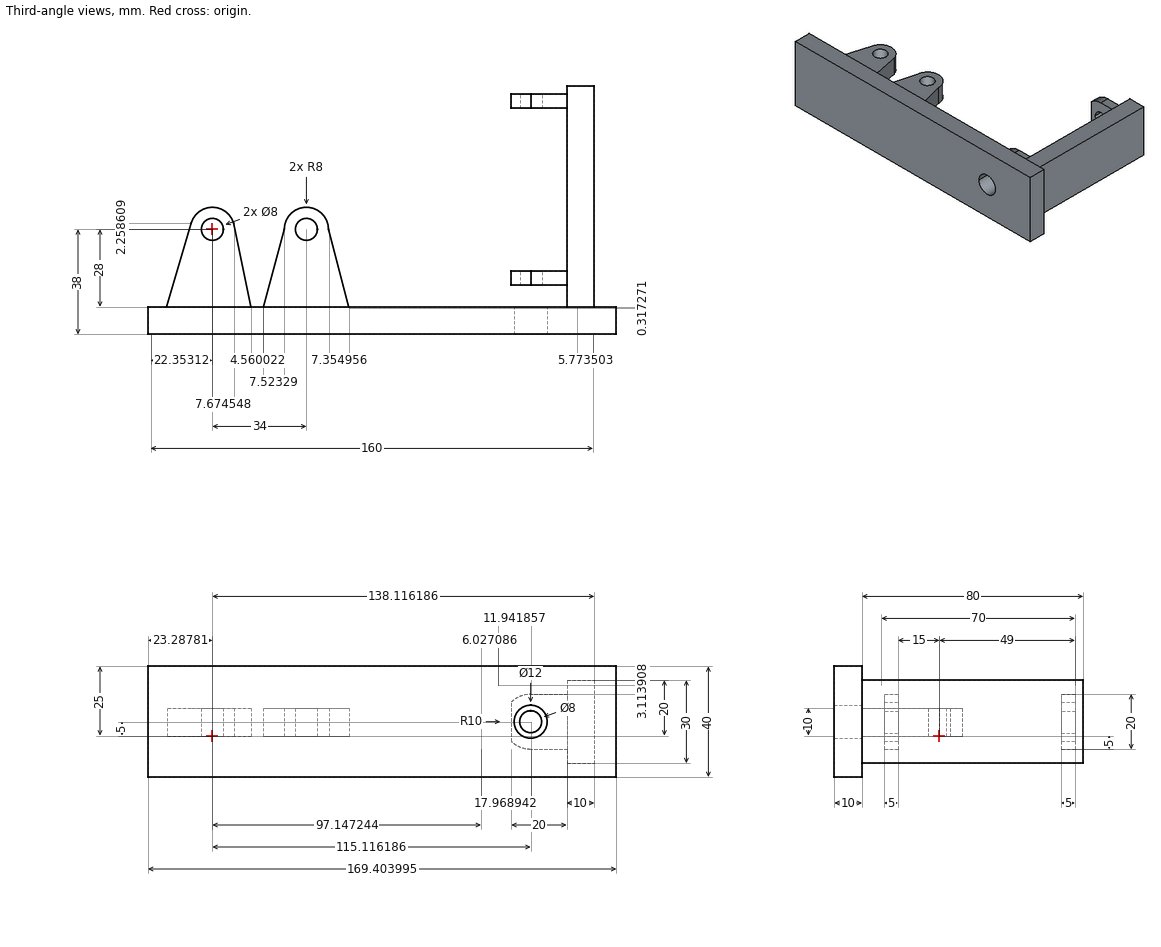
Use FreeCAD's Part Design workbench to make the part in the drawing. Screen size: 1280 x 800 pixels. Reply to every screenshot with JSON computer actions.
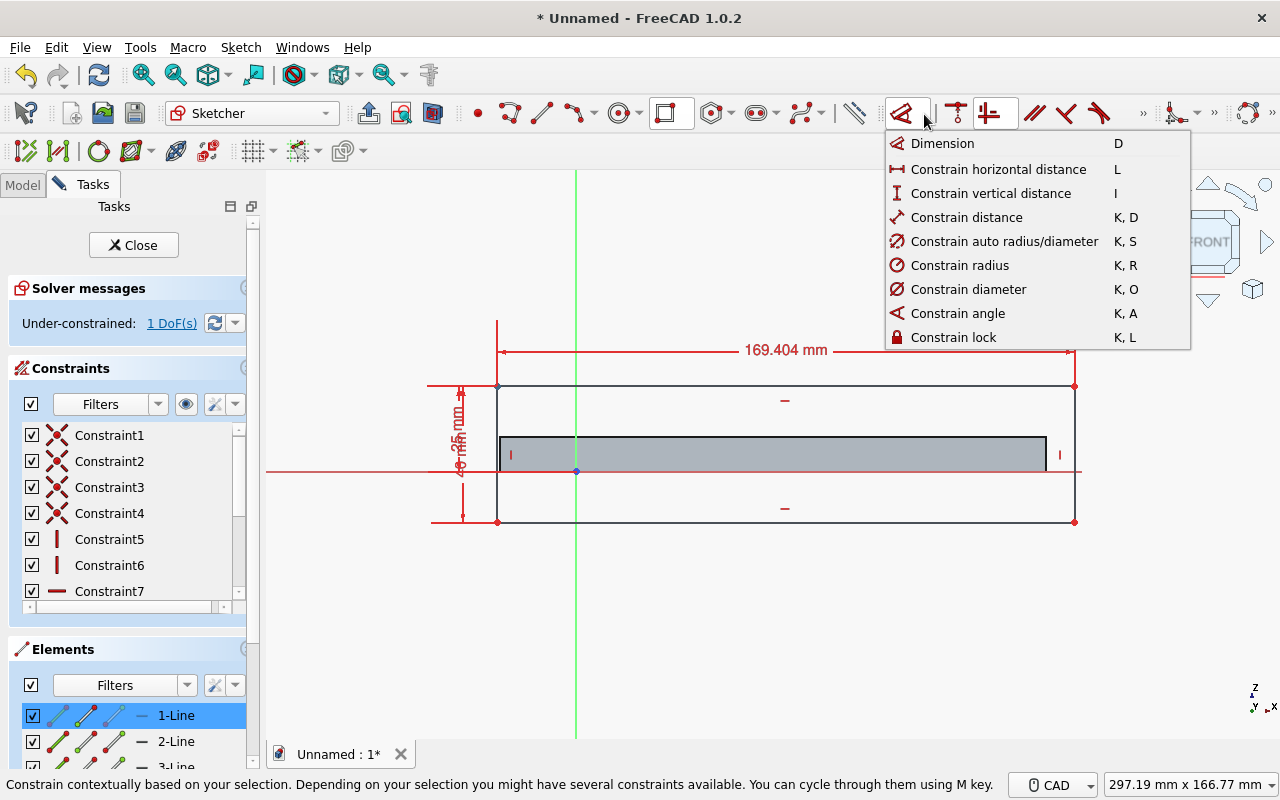
{"action": "left_click", "coordinate": [1038, 169]}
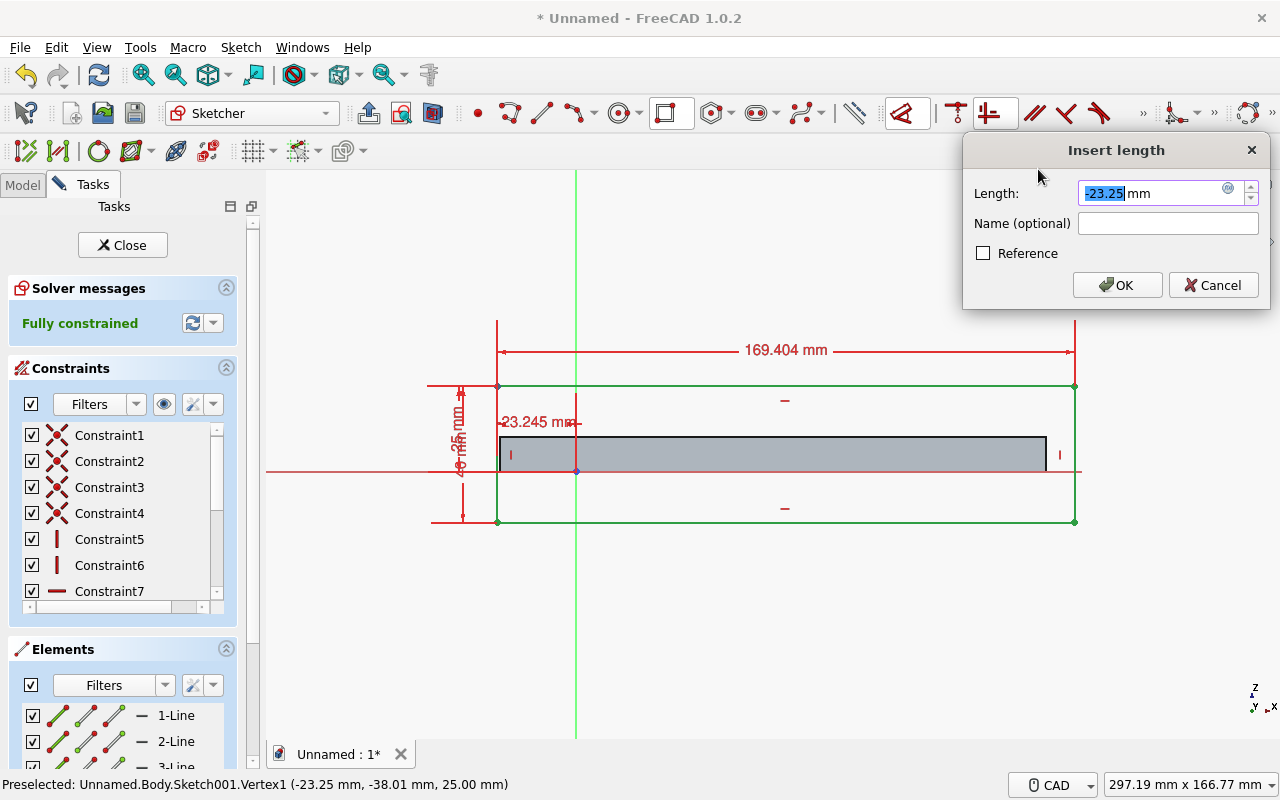
{"action": "type", "text": "-23.28781"}
{"action": "key", "text": "Return"}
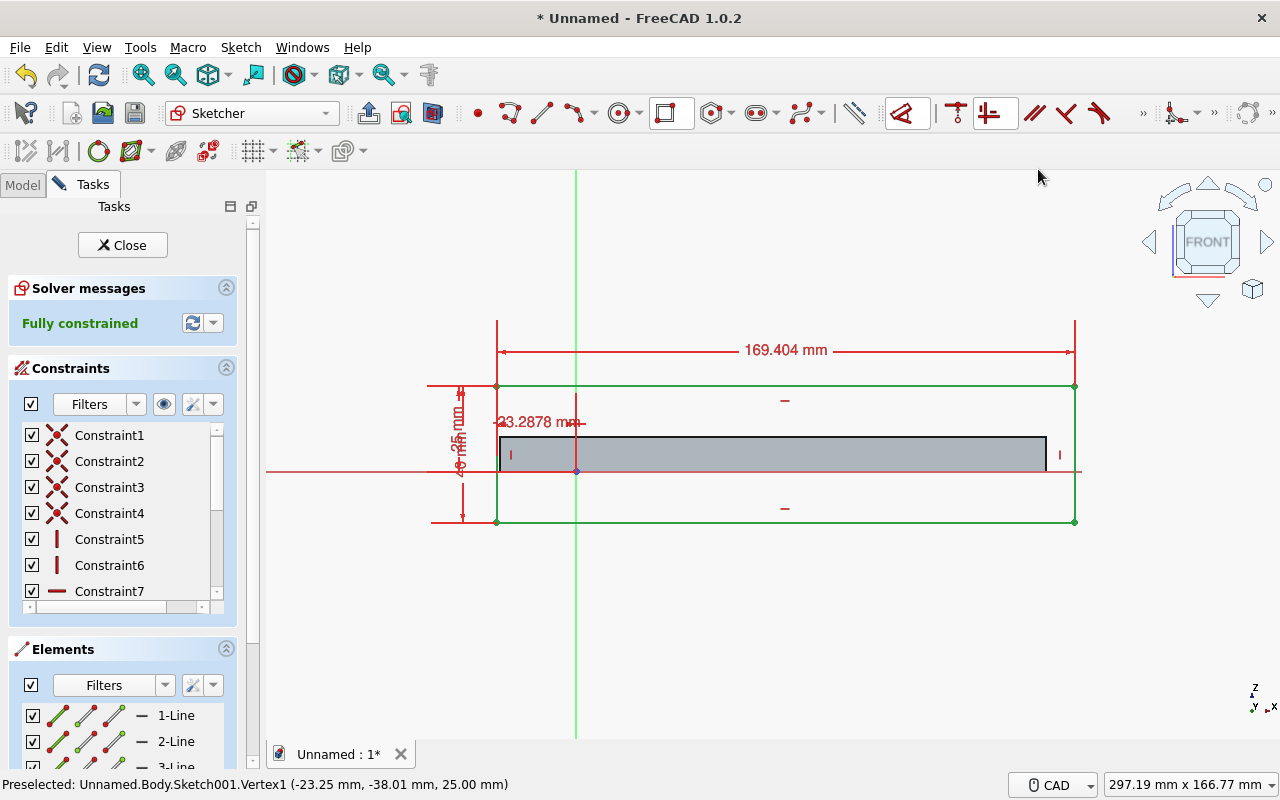
{"action": "left_click", "coordinate": [123, 245]}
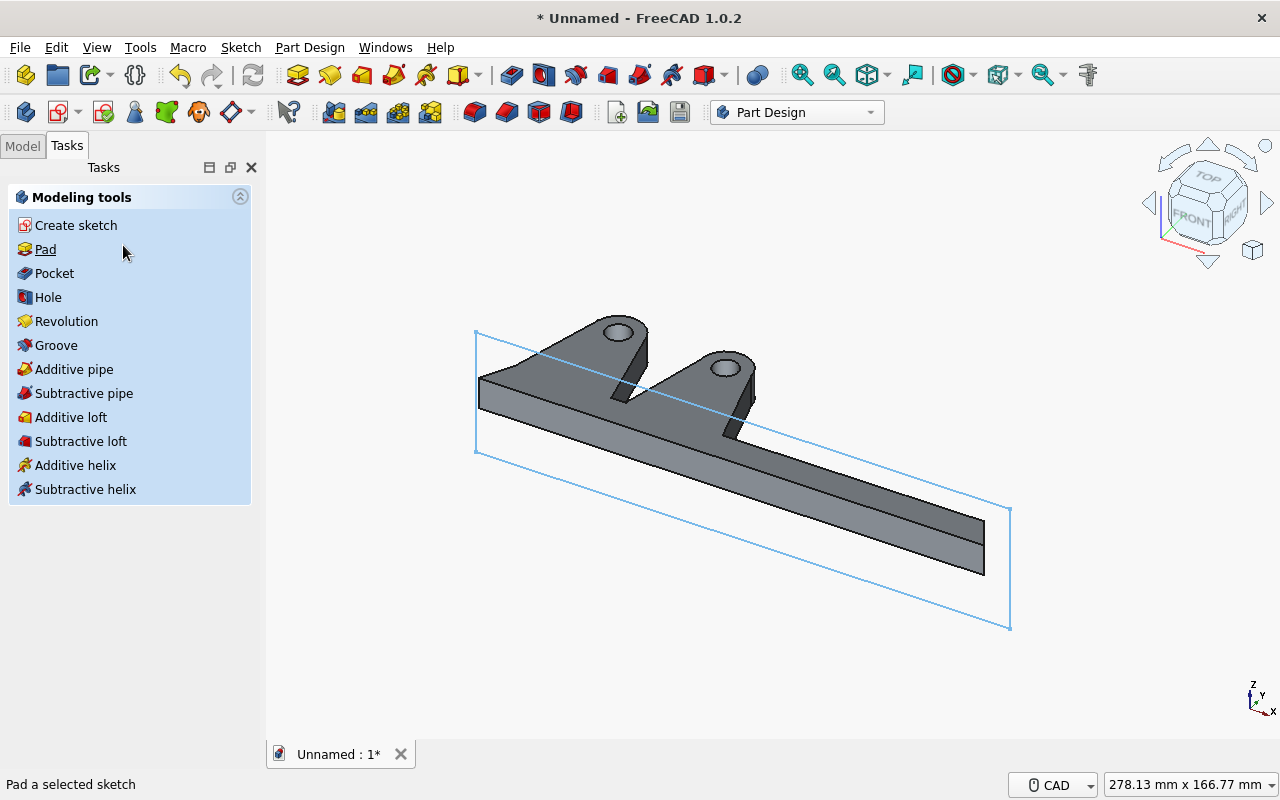
{"action": "left_click", "coordinate": [298, 76]}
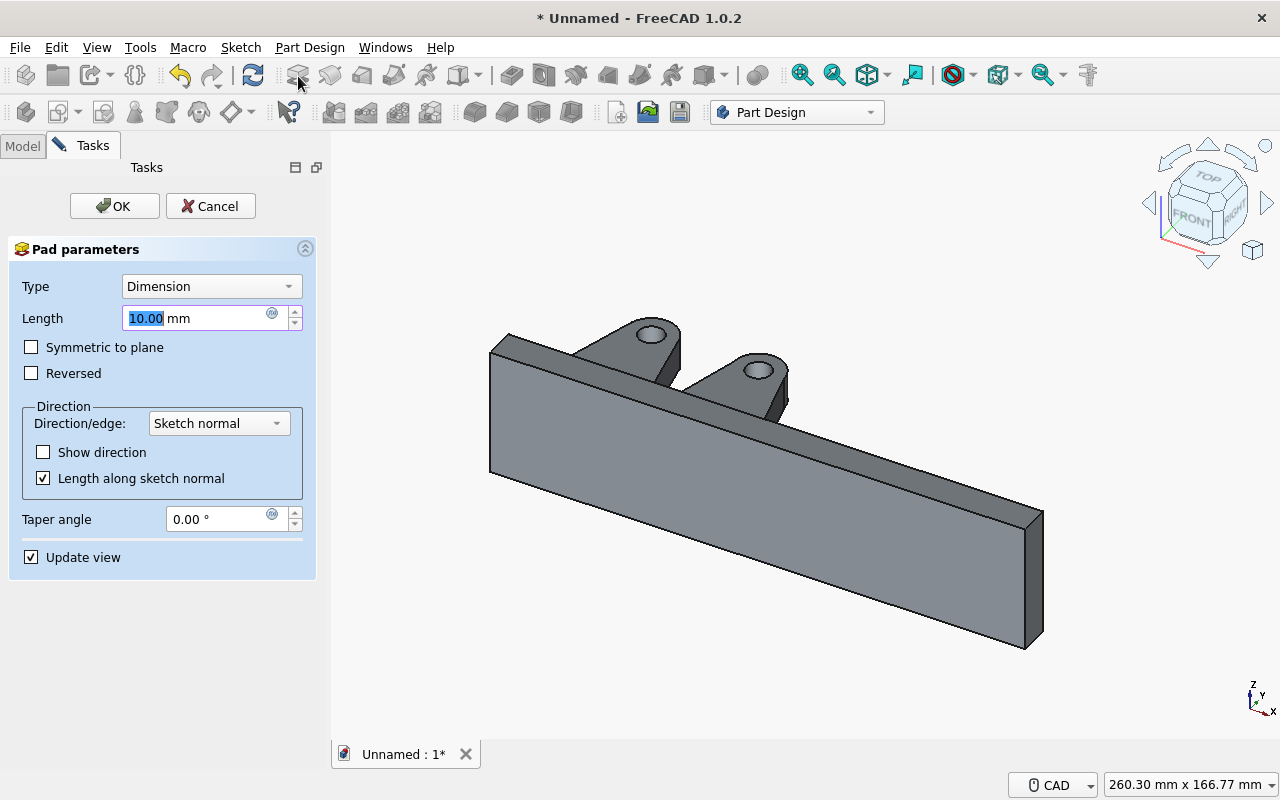
{"action": "type", "text": "10"}
{"action": "key", "text": "Tab"}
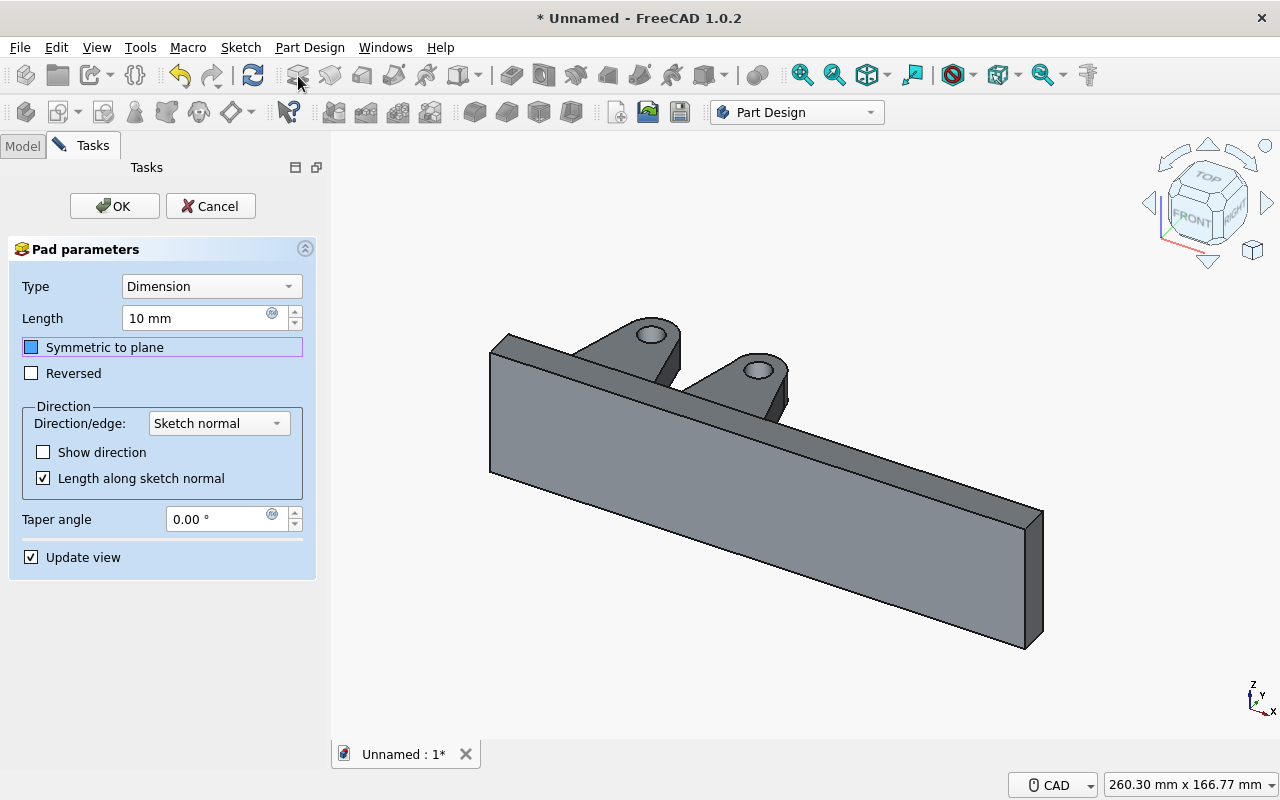
{"action": "left_click", "coordinate": [30, 373]}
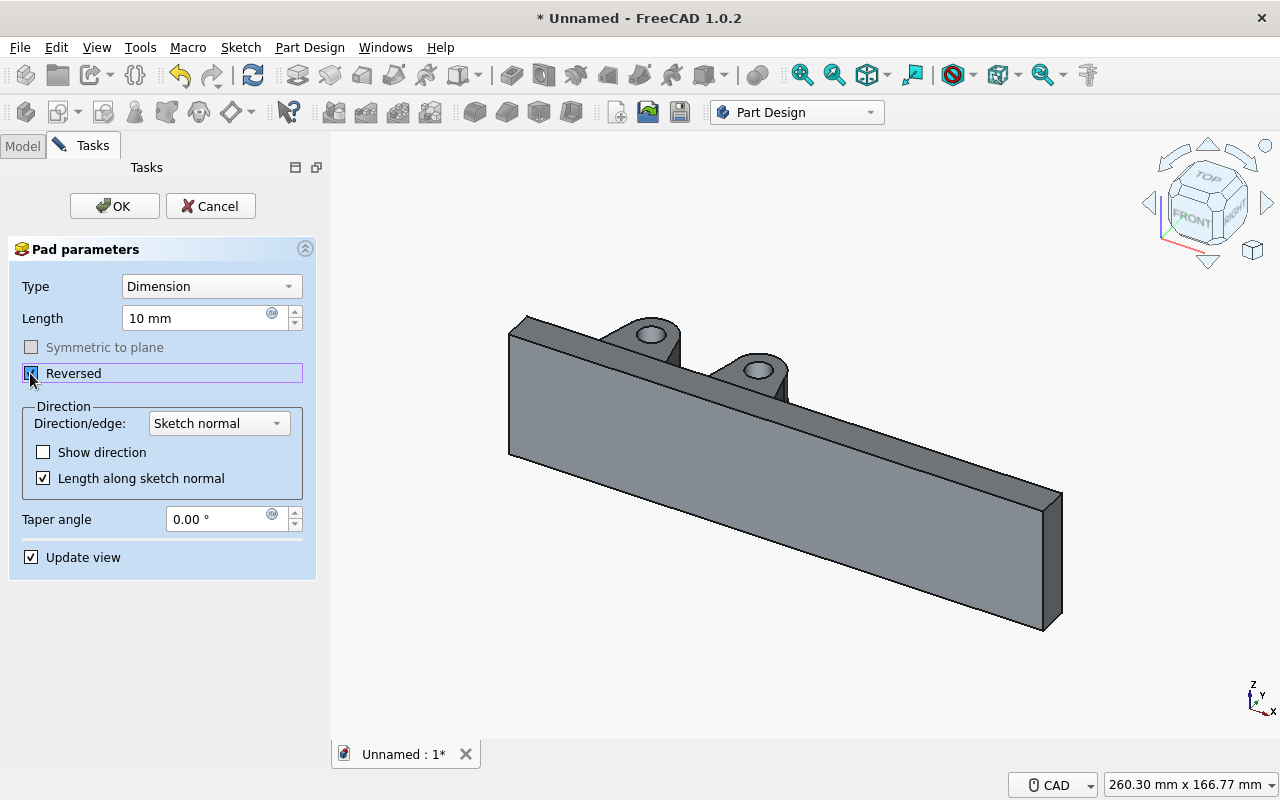
{"action": "left_click", "coordinate": [115, 206]}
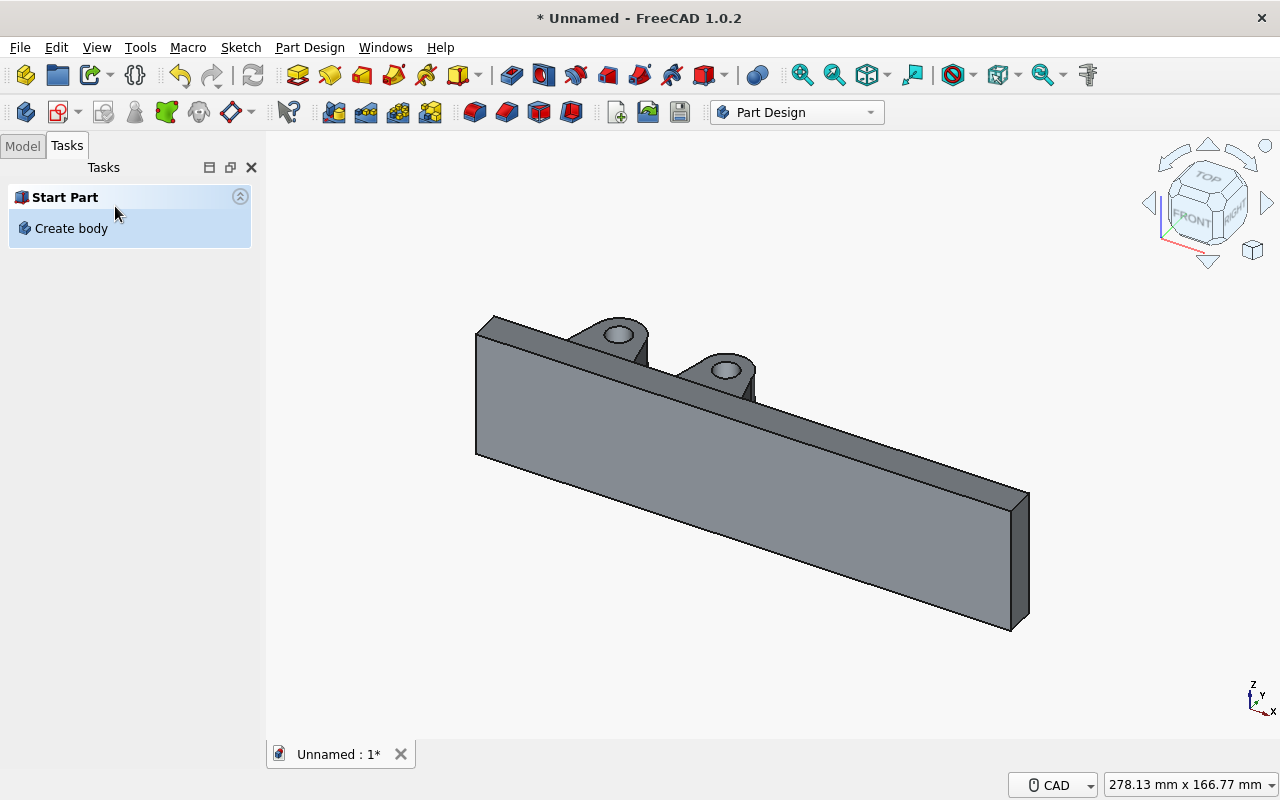
{"action": "key", "text": "4"}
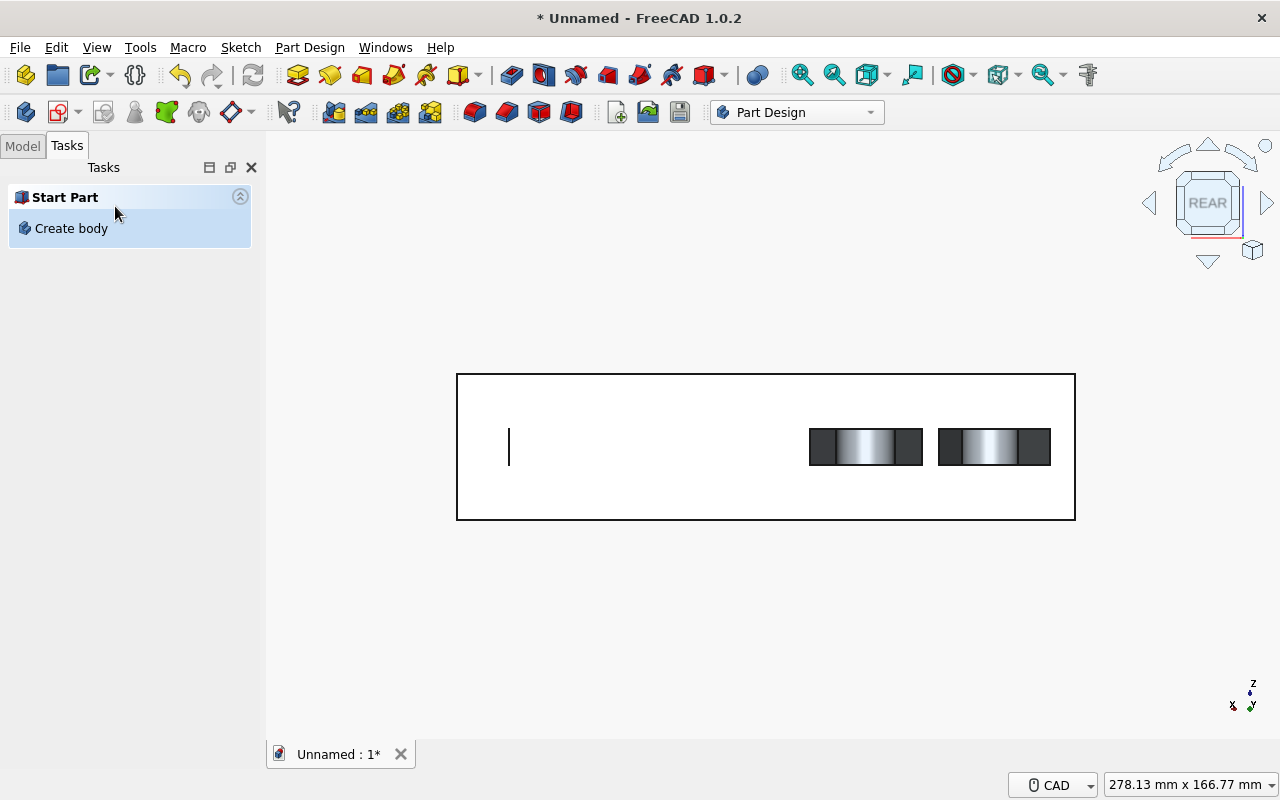
{"action": "left_click", "coordinate": [589, 446]}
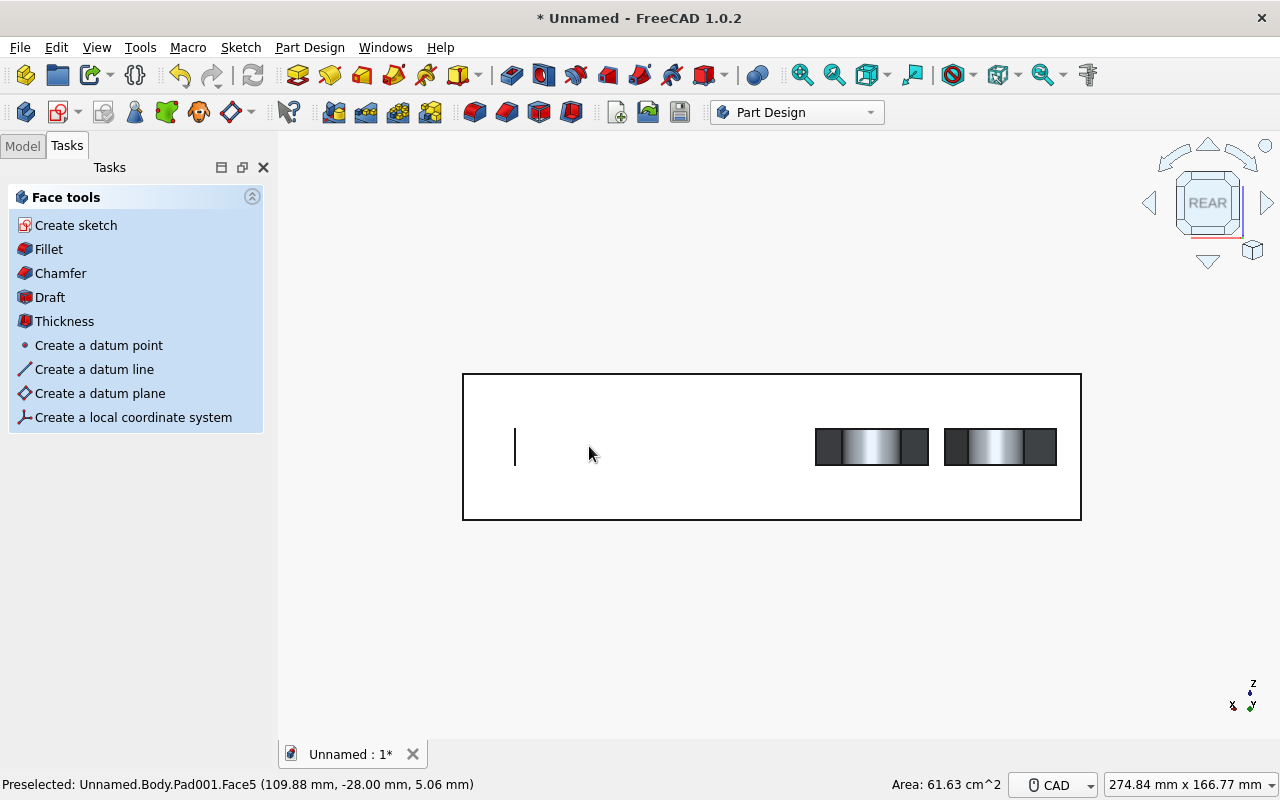
{"action": "left_click", "coordinate": [58, 112]}